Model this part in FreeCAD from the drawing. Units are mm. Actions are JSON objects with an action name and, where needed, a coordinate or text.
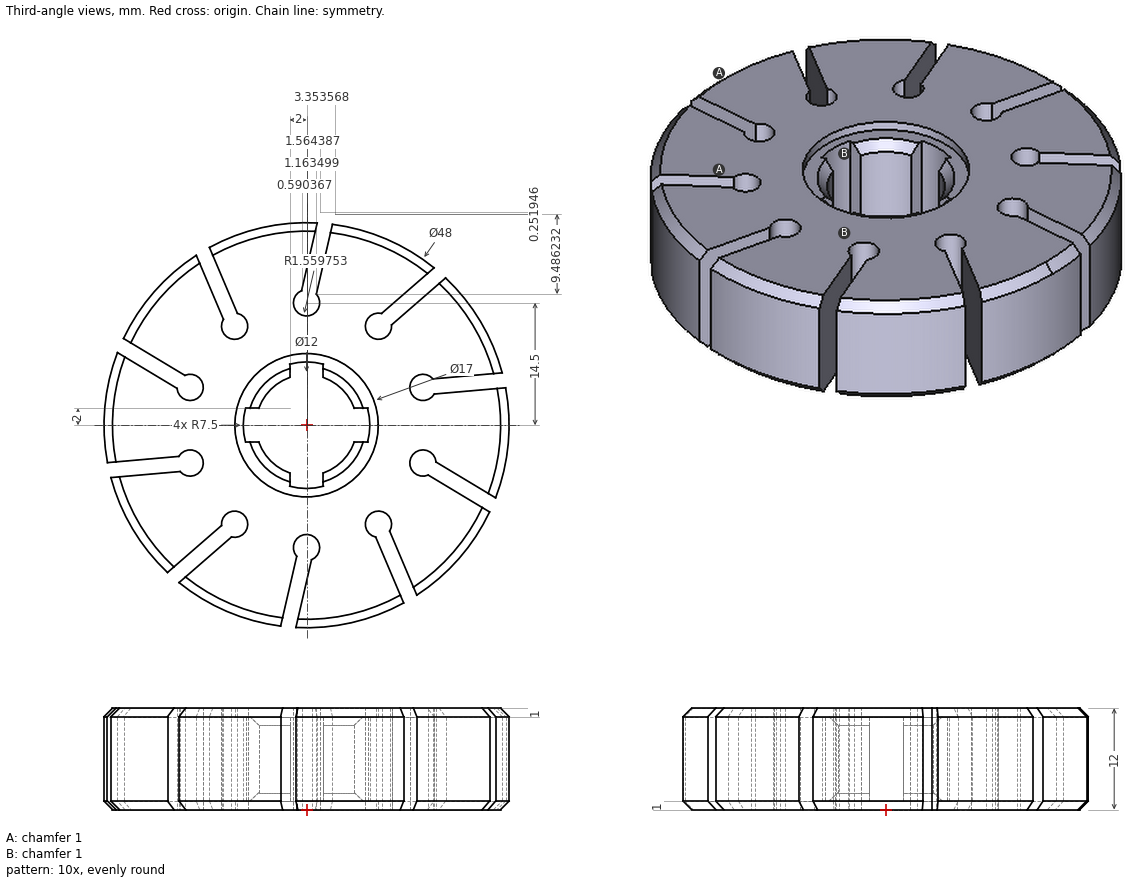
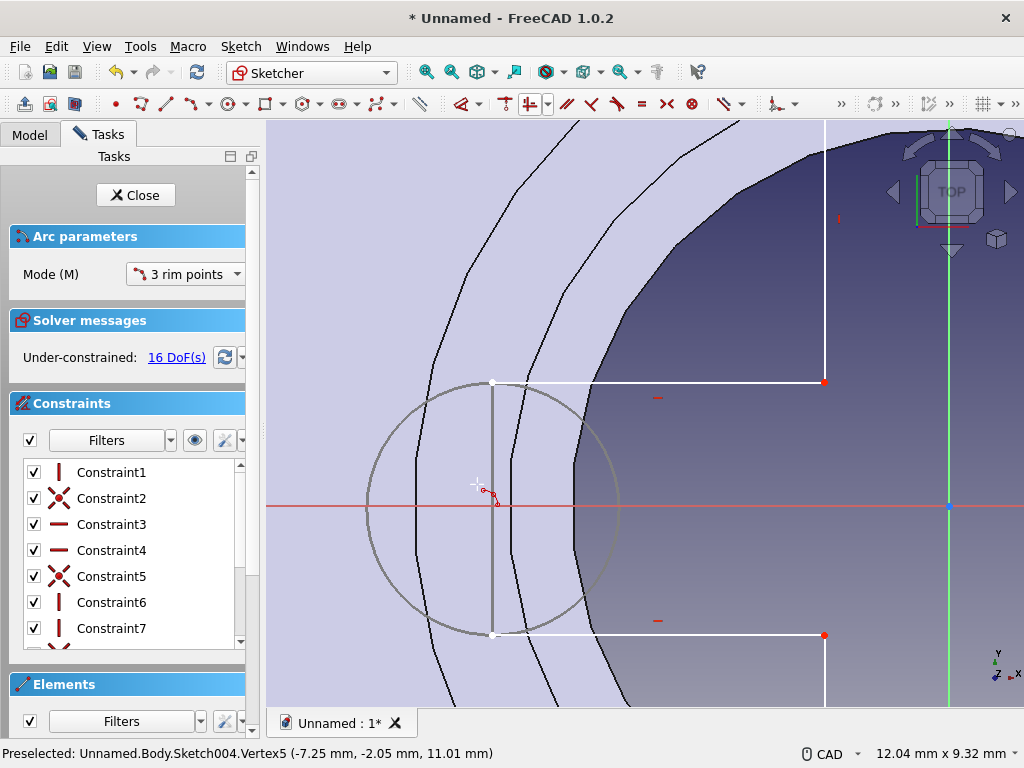
{"action": "left_click", "coordinate": [478, 481]}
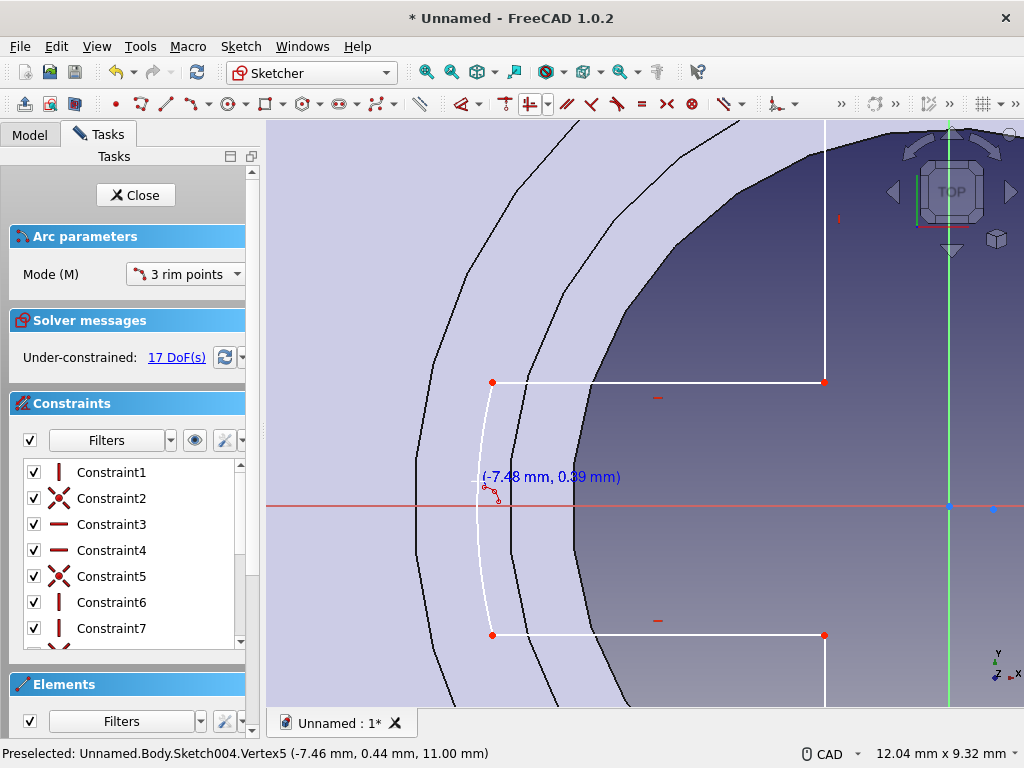
{"action": "scroll", "coordinate": [360, 359], "scroll_direction": "down", "scroll_amount": 5}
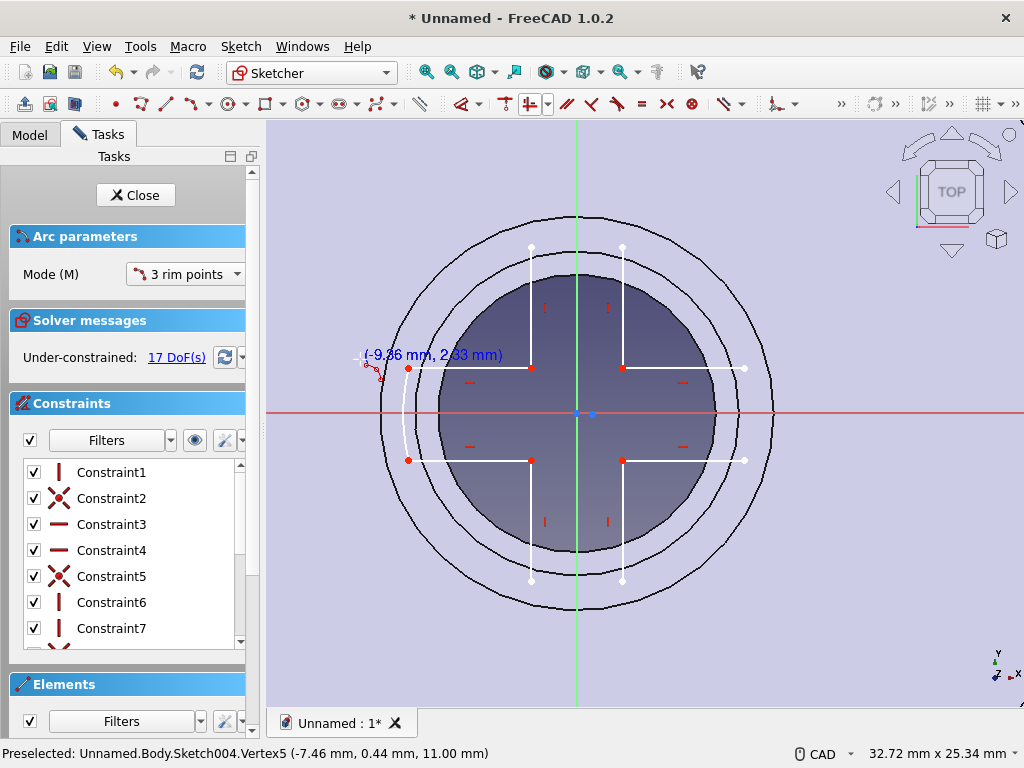
{"action": "left_click", "coordinate": [531, 582]}
{"action": "left_click", "coordinate": [623, 582]}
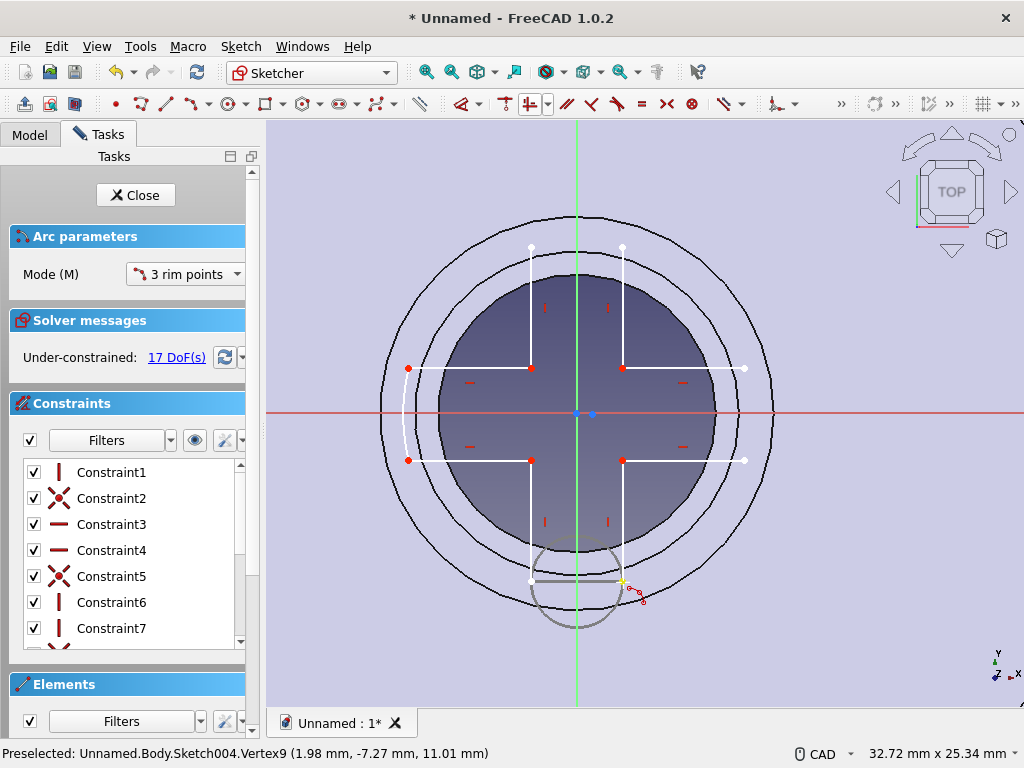
{"action": "scroll", "coordinate": [567, 587], "scroll_direction": "up", "scroll_amount": 5}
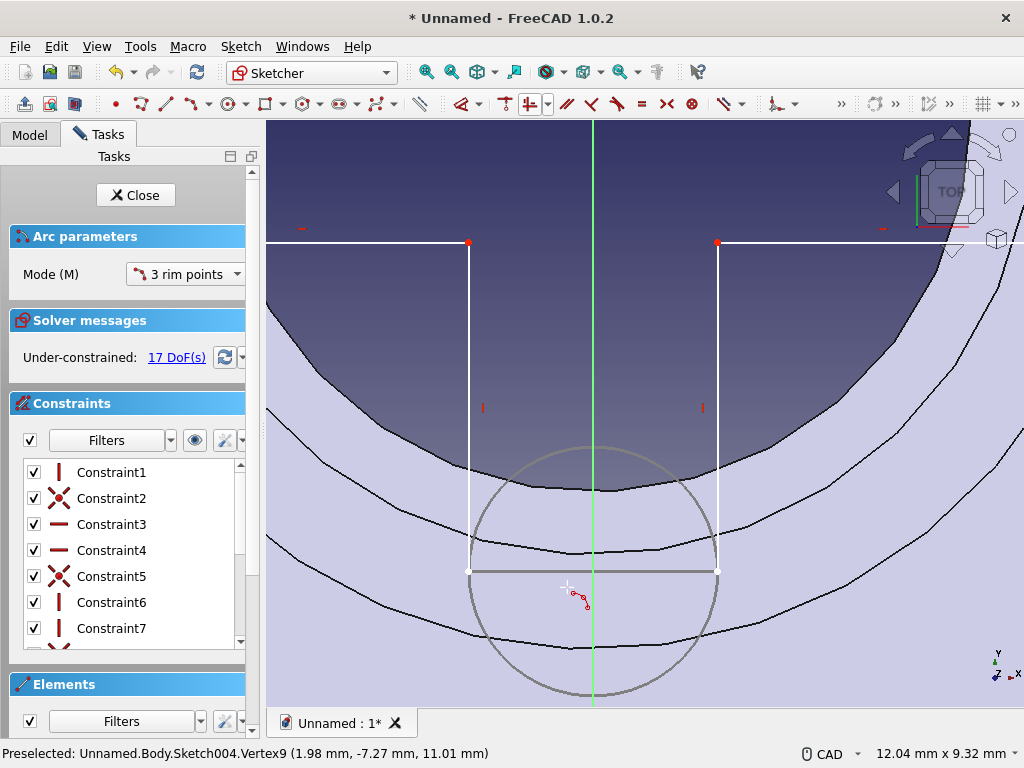
{"action": "left_click", "coordinate": [568, 586]}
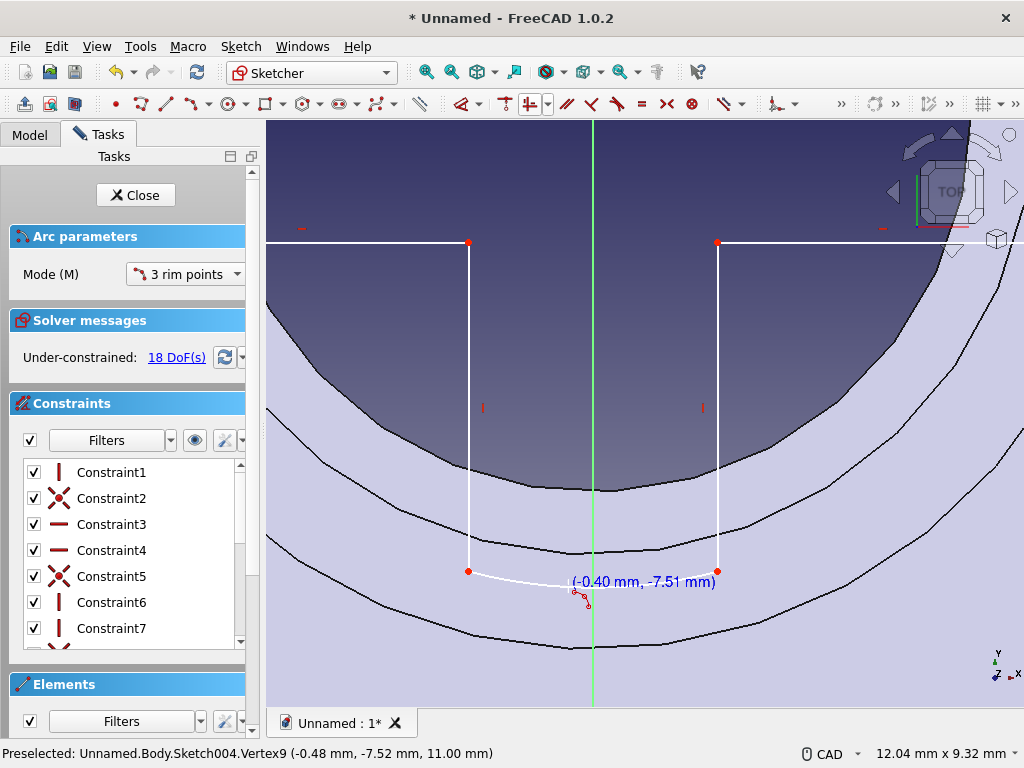
{"action": "scroll", "coordinate": [567, 588], "scroll_direction": "down", "scroll_amount": 5}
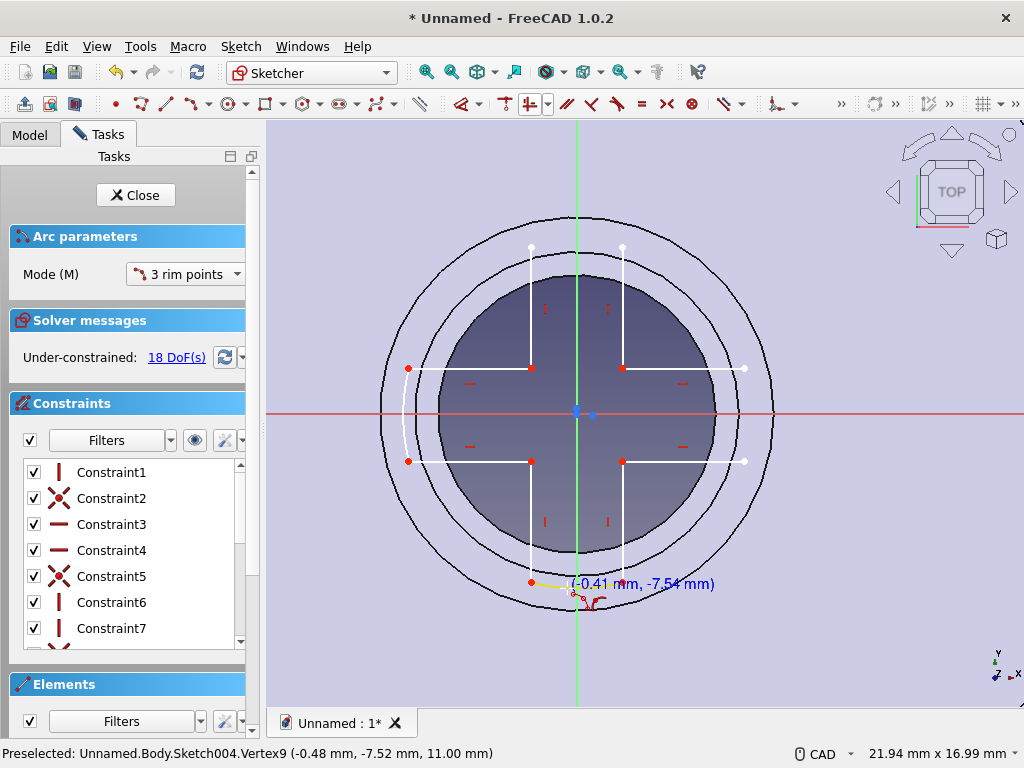
{"action": "left_click", "coordinate": [745, 462]}
{"action": "left_click", "coordinate": [745, 369]}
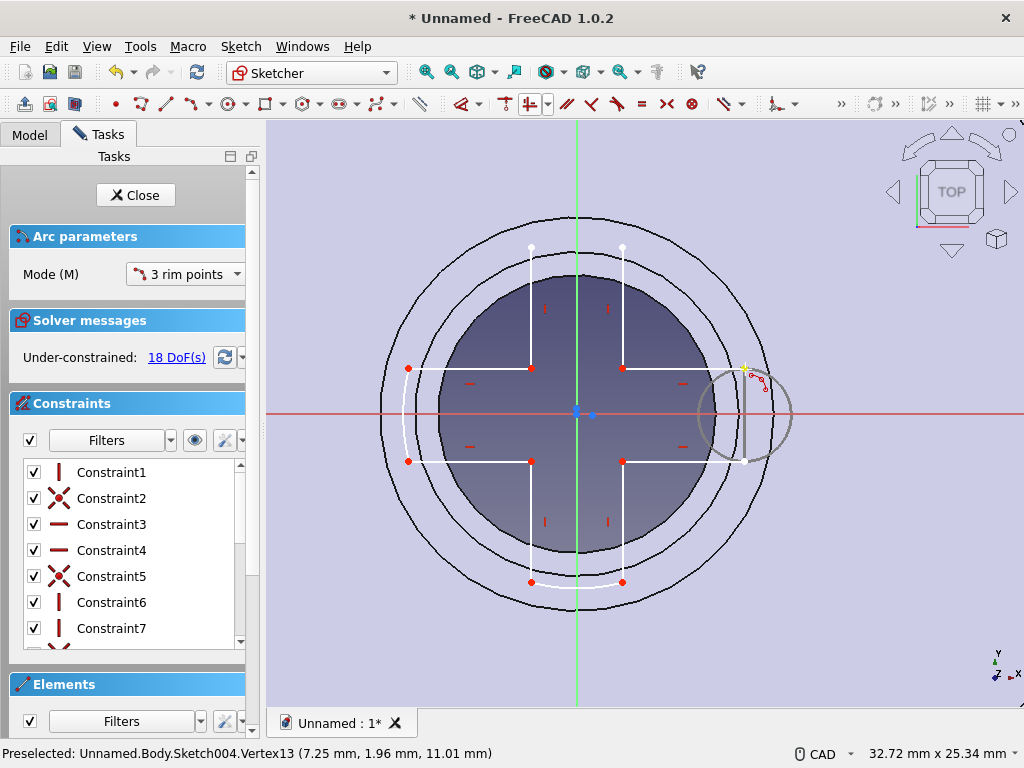
{"action": "scroll", "coordinate": [750, 424], "scroll_direction": "up", "scroll_amount": 5}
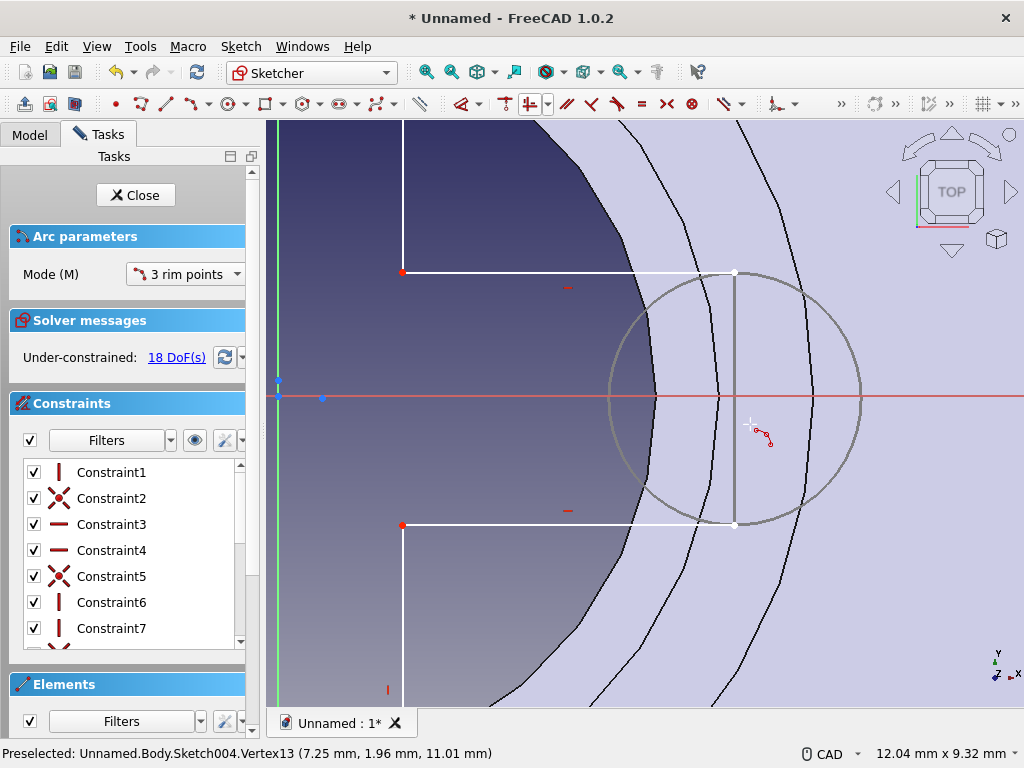
{"action": "left_click", "coordinate": [750, 422]}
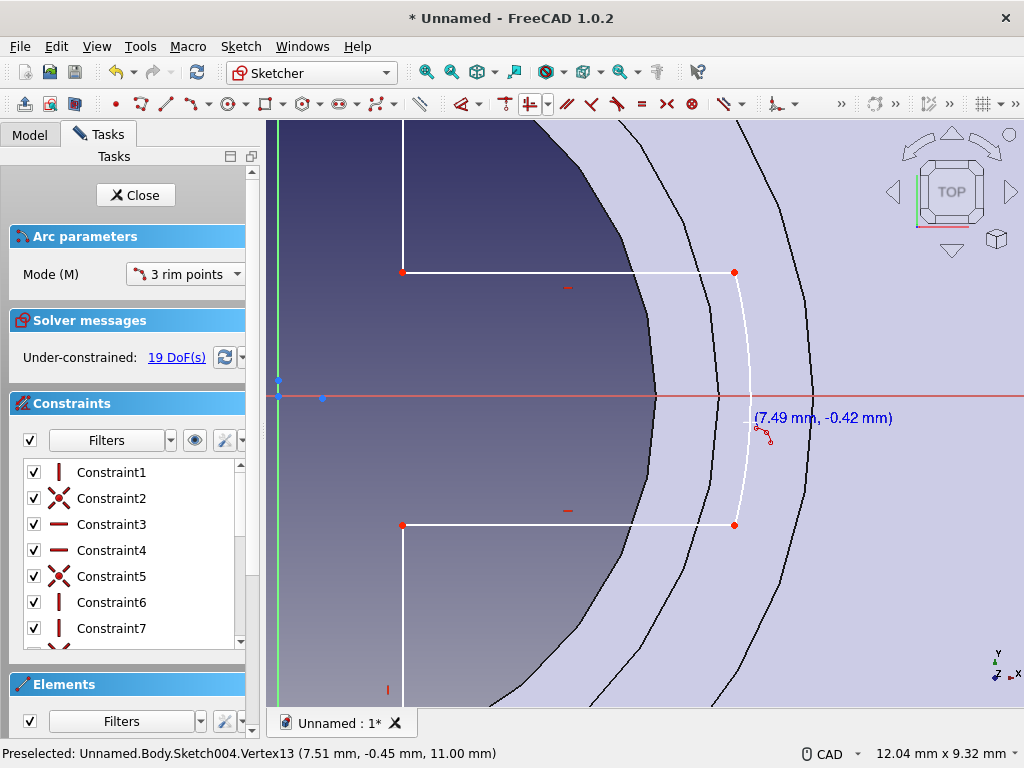
{"action": "scroll", "coordinate": [750, 424], "scroll_direction": "down", "scroll_amount": 5}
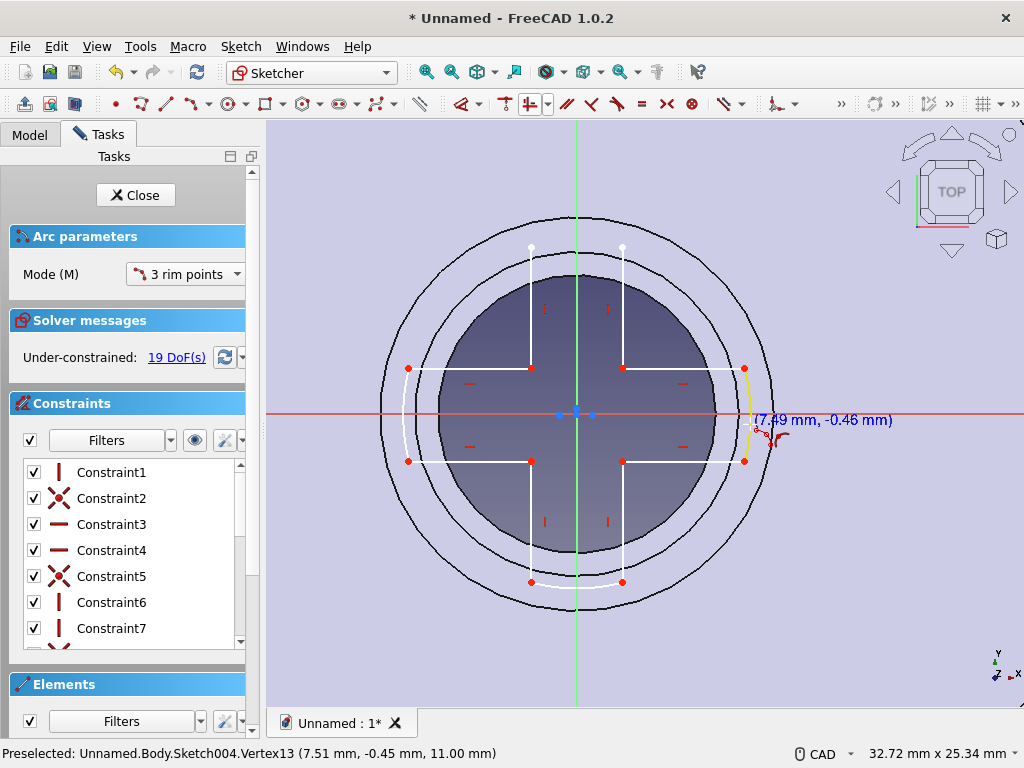
{"action": "left_click", "coordinate": [623, 248]}
{"action": "left_click", "coordinate": [531, 248]}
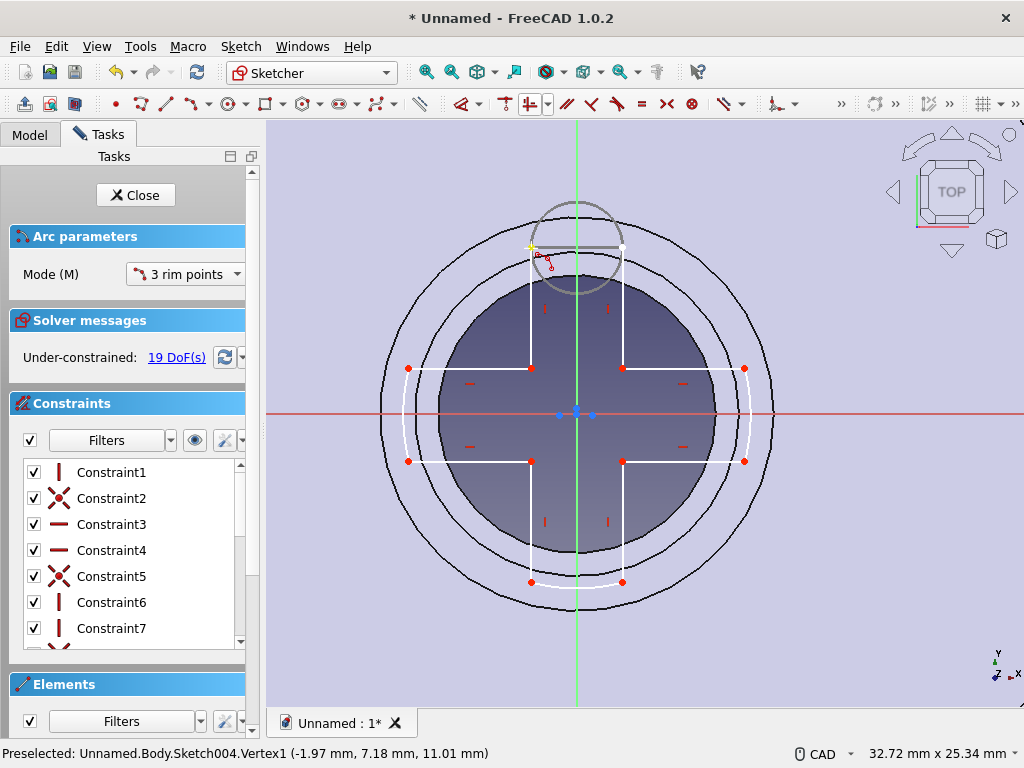
{"action": "scroll", "coordinate": [586, 241], "scroll_direction": "up", "scroll_amount": 5}